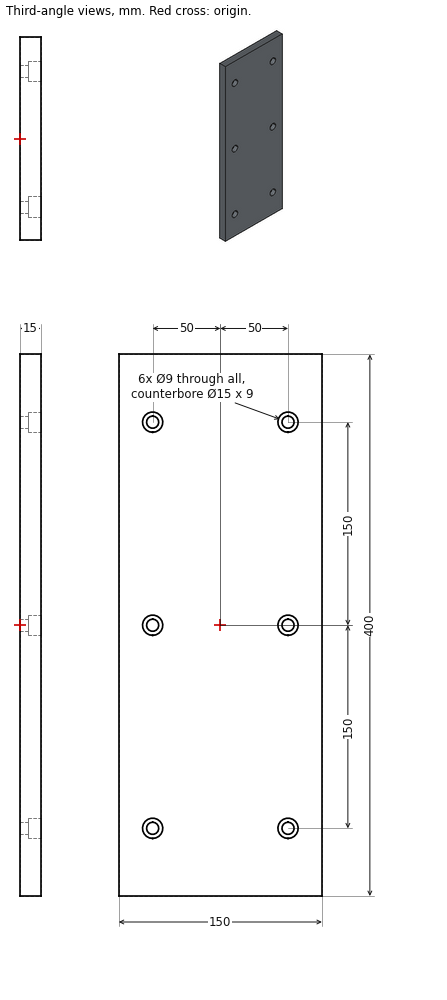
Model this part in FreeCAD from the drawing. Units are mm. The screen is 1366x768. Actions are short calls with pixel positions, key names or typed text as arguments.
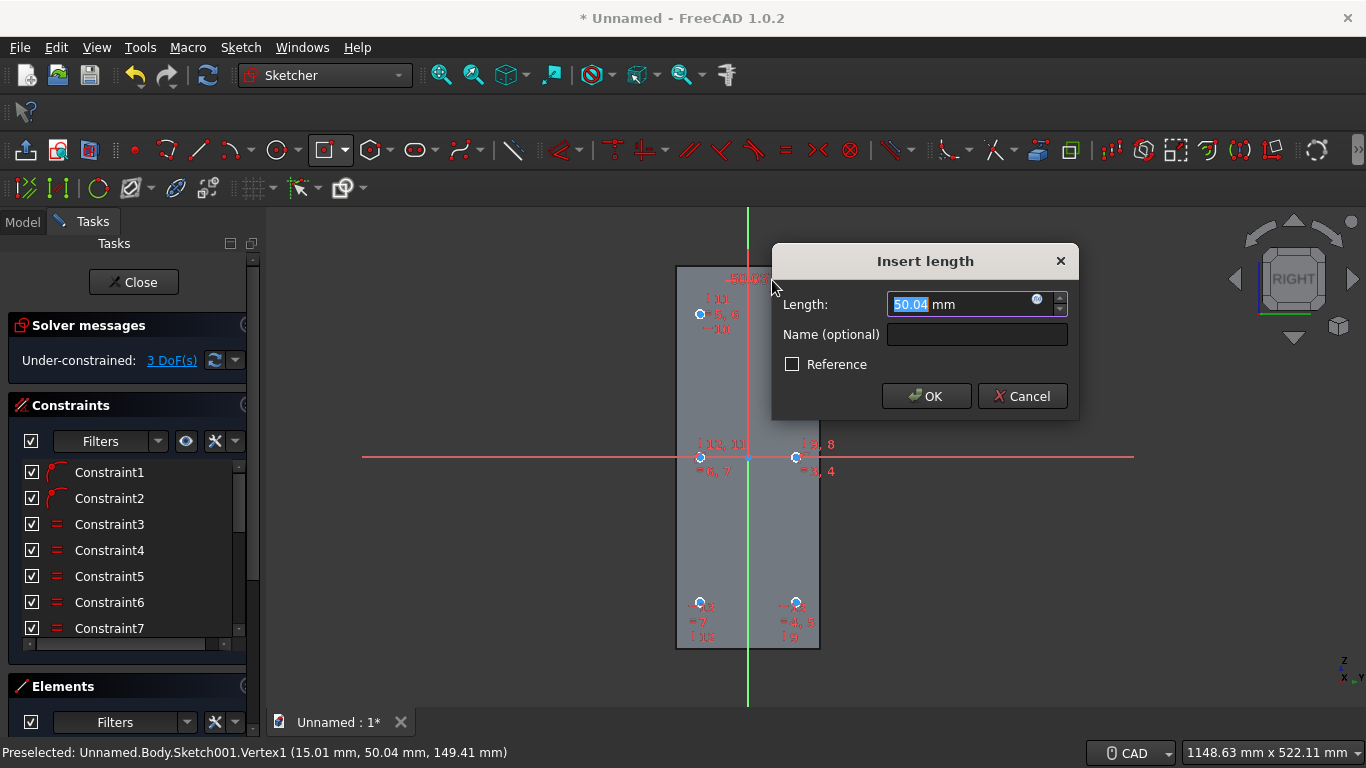
text(50)
key(Return)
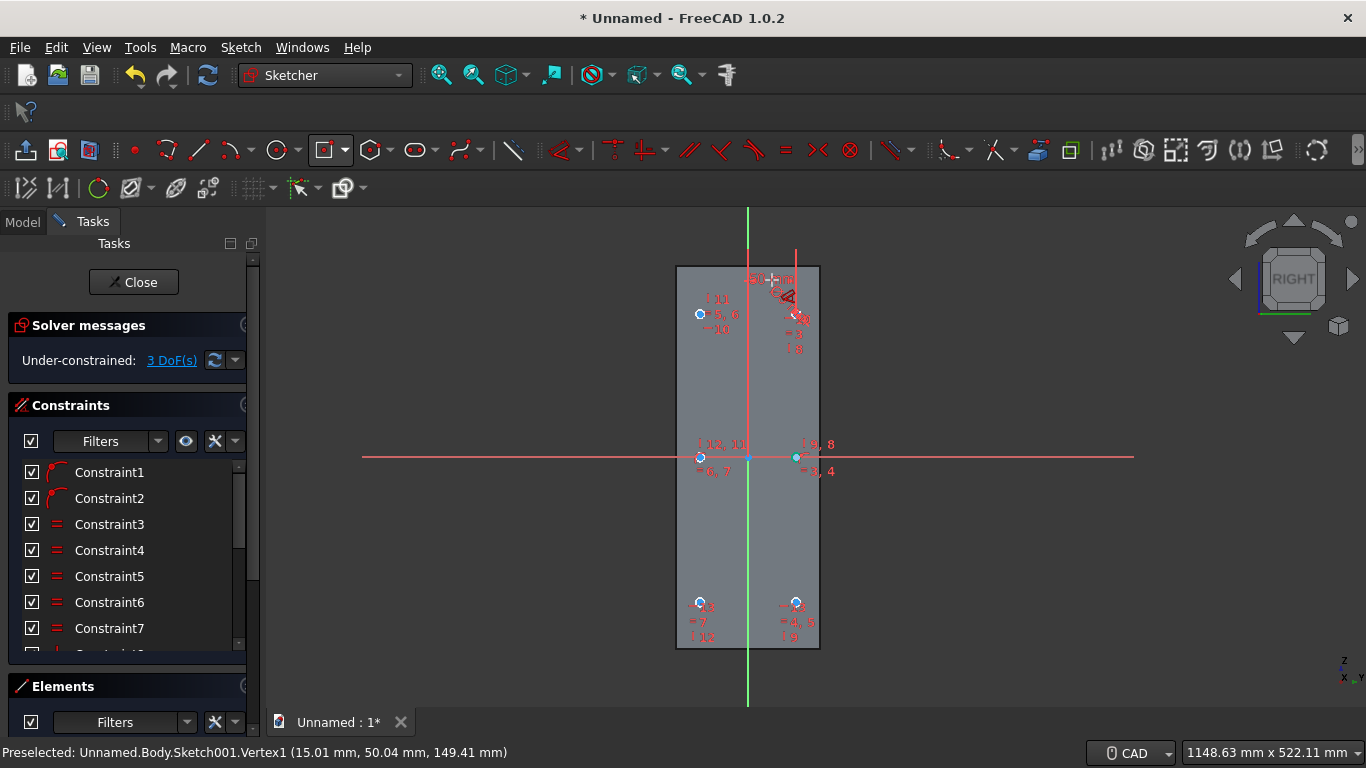
click(700, 314)
click(724, 491)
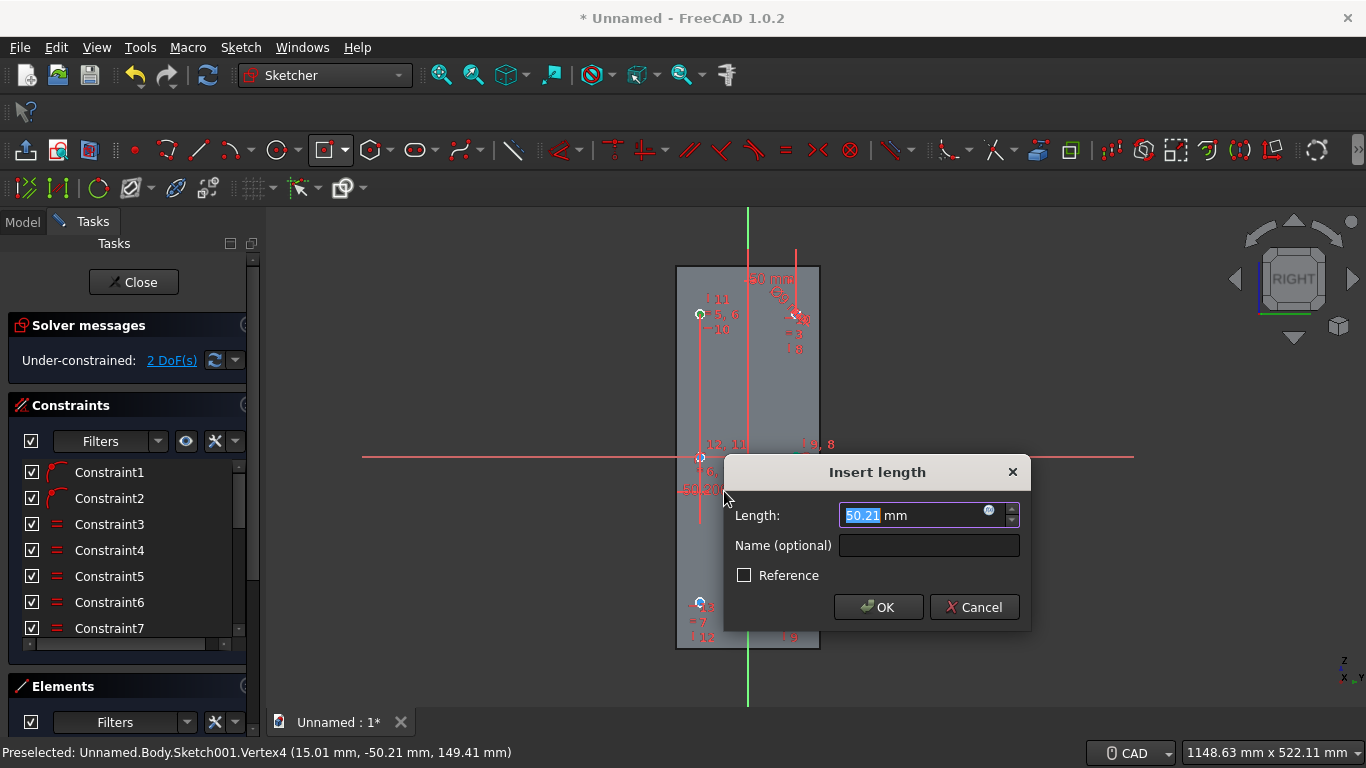
text(50)
key(Return)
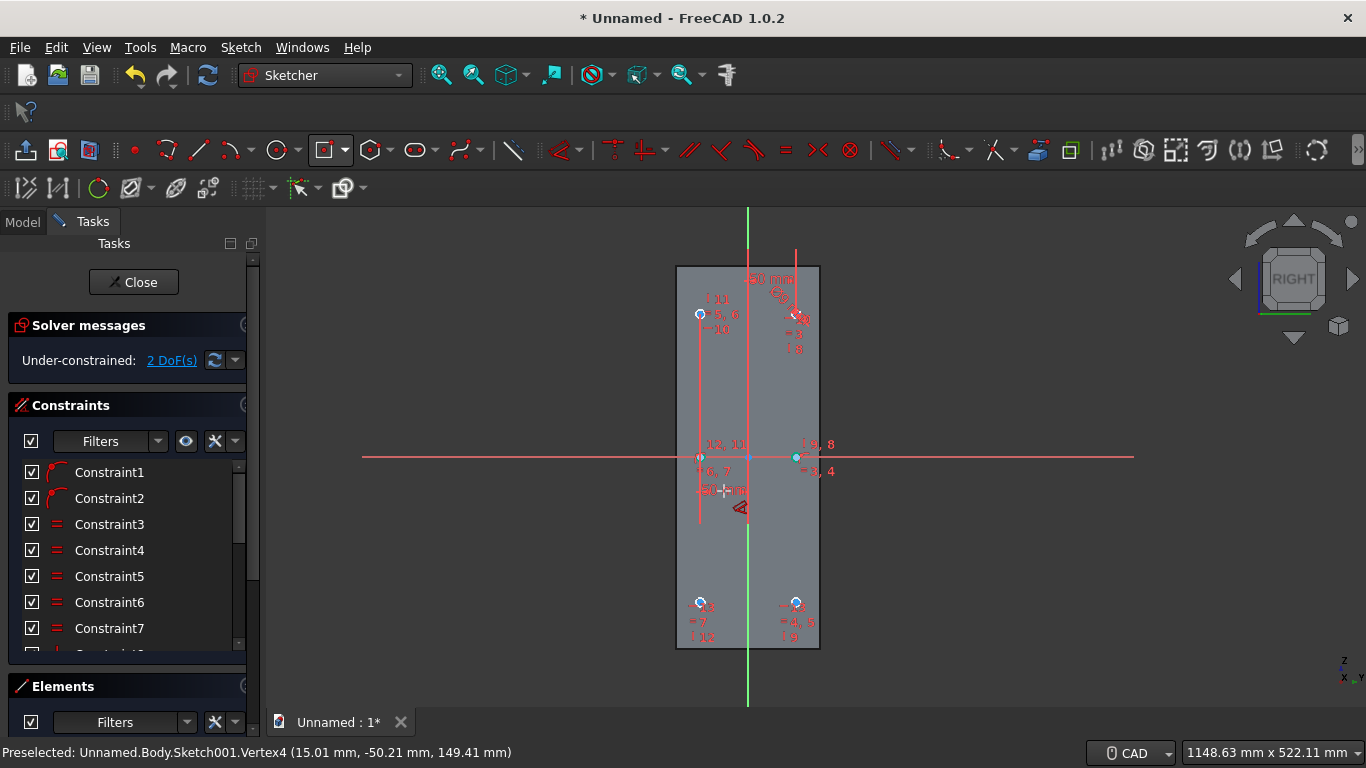
click(796, 314)
click(830, 386)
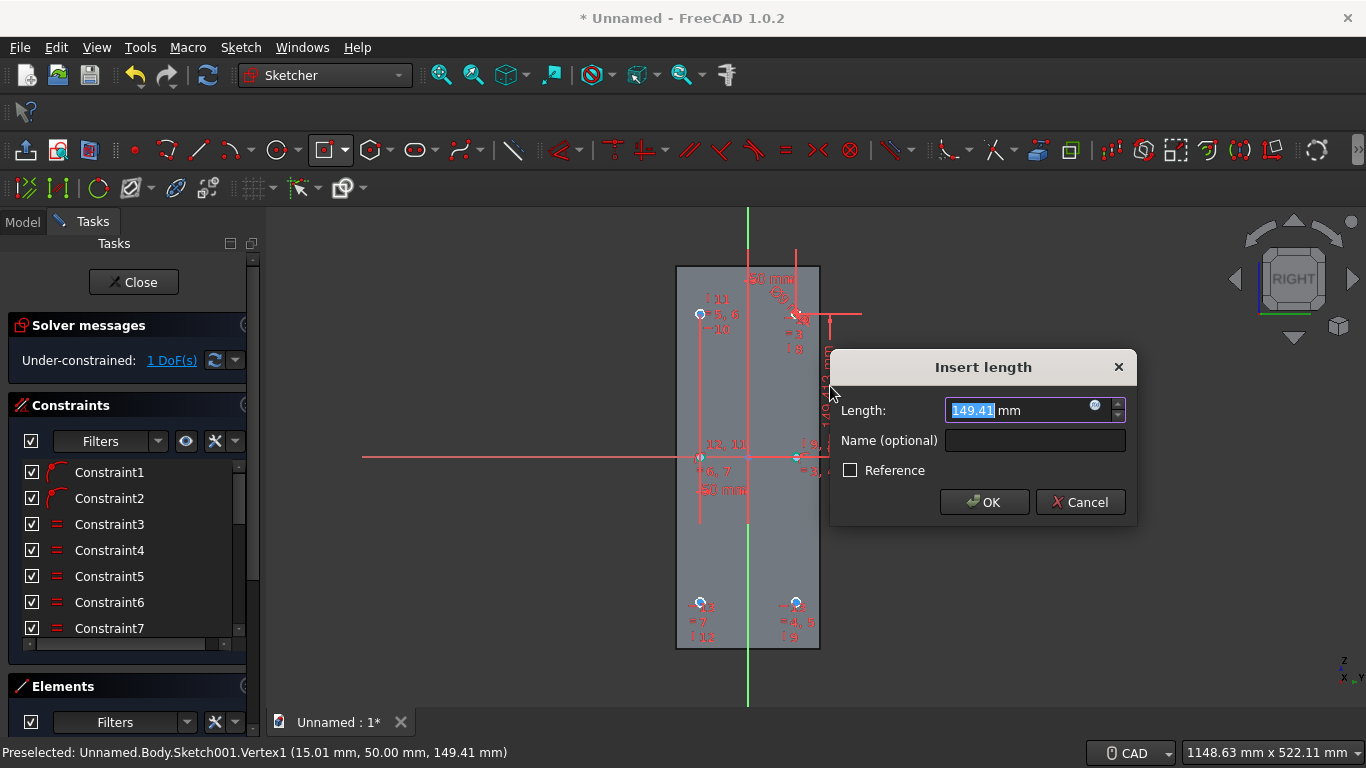
text(150)
key(Return)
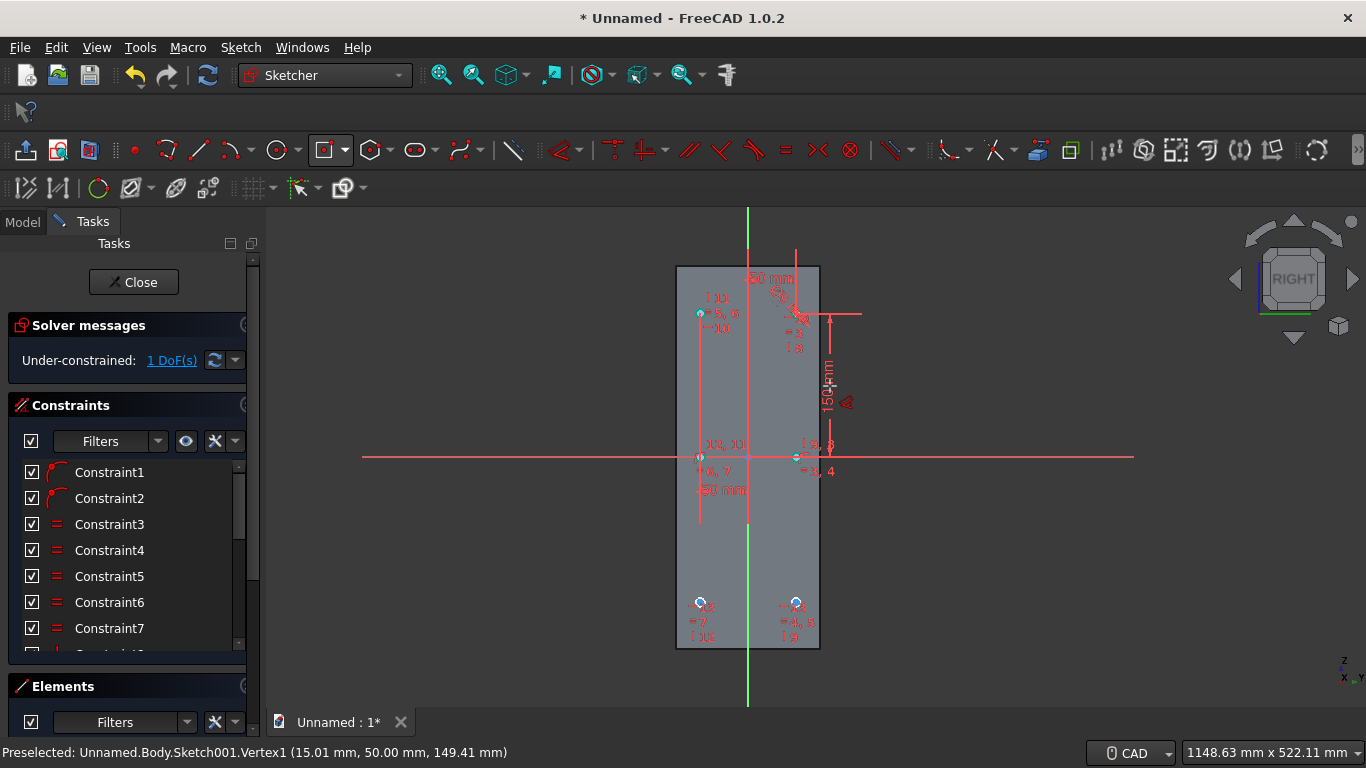
click(796, 602)
click(830, 530)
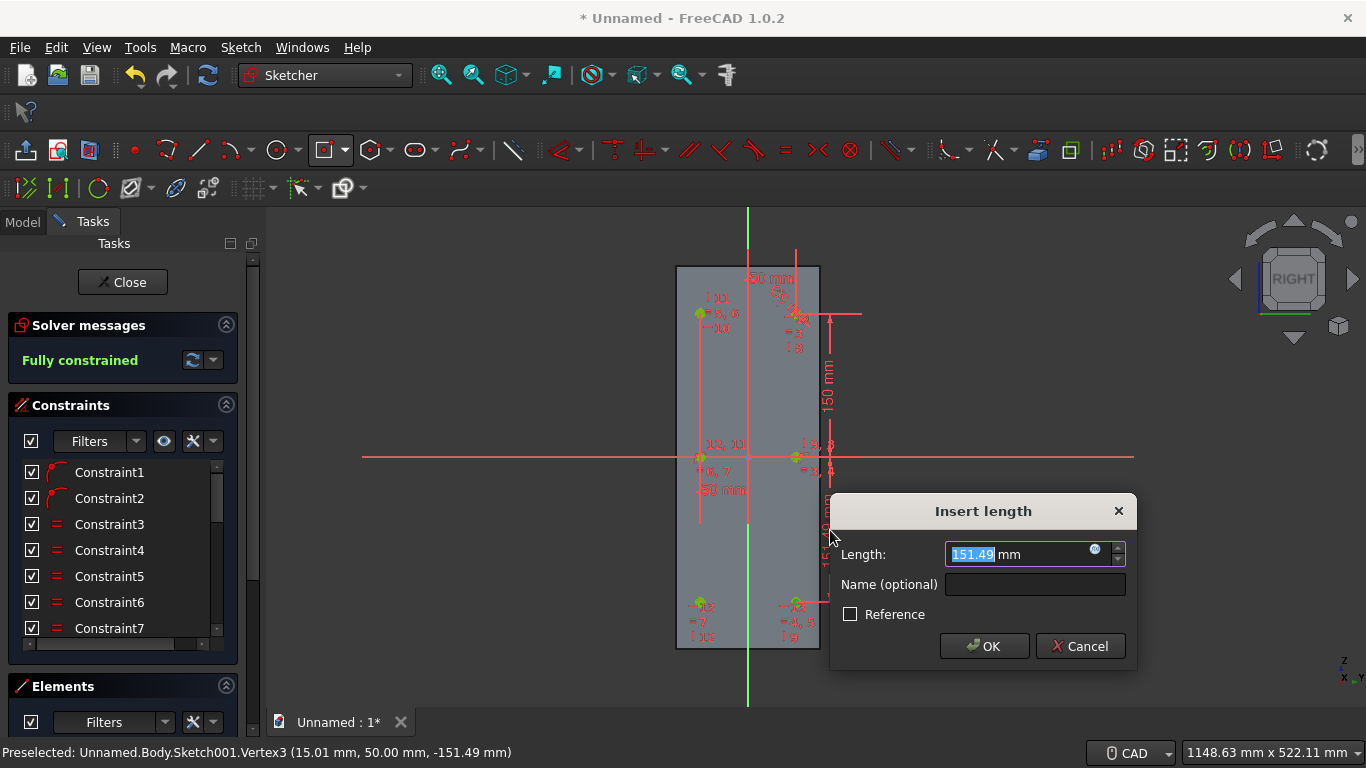
text(150)
key(Return)
key(Escape)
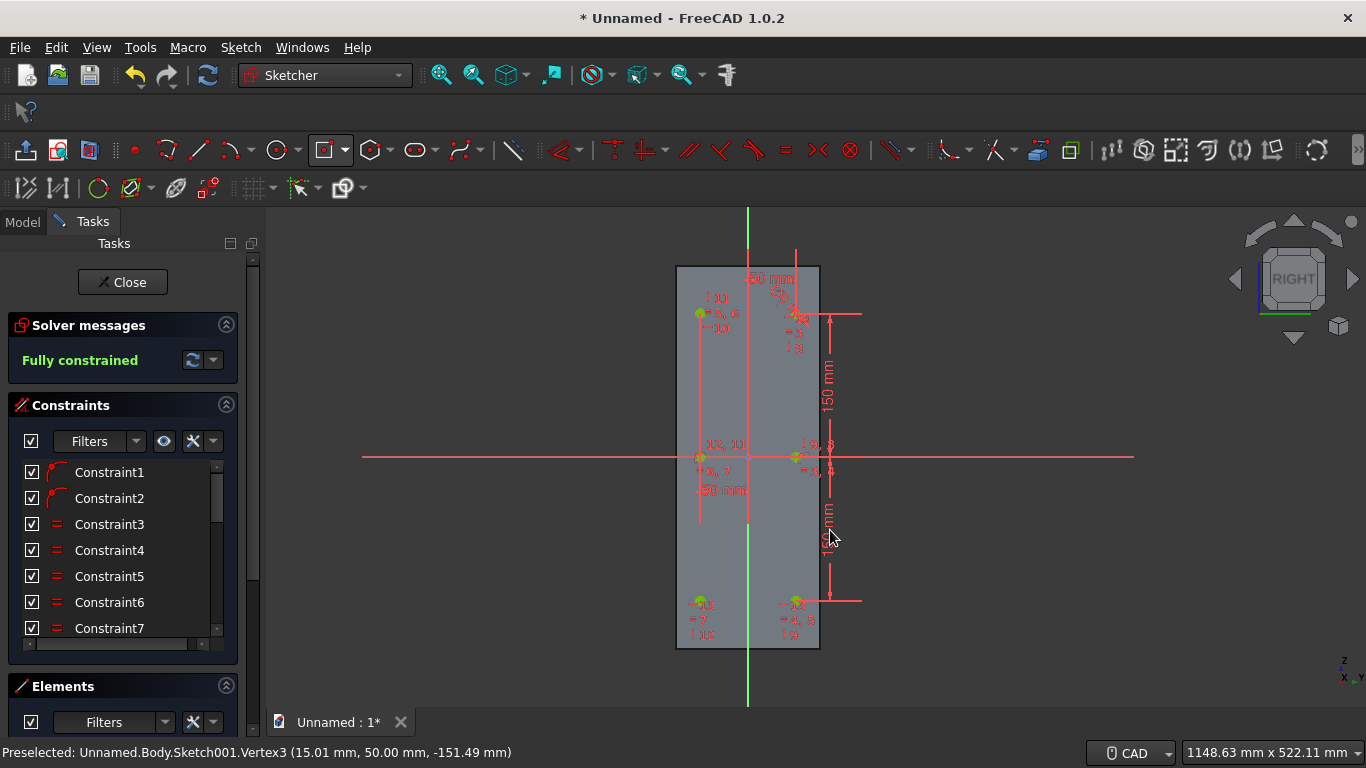
click(123, 282)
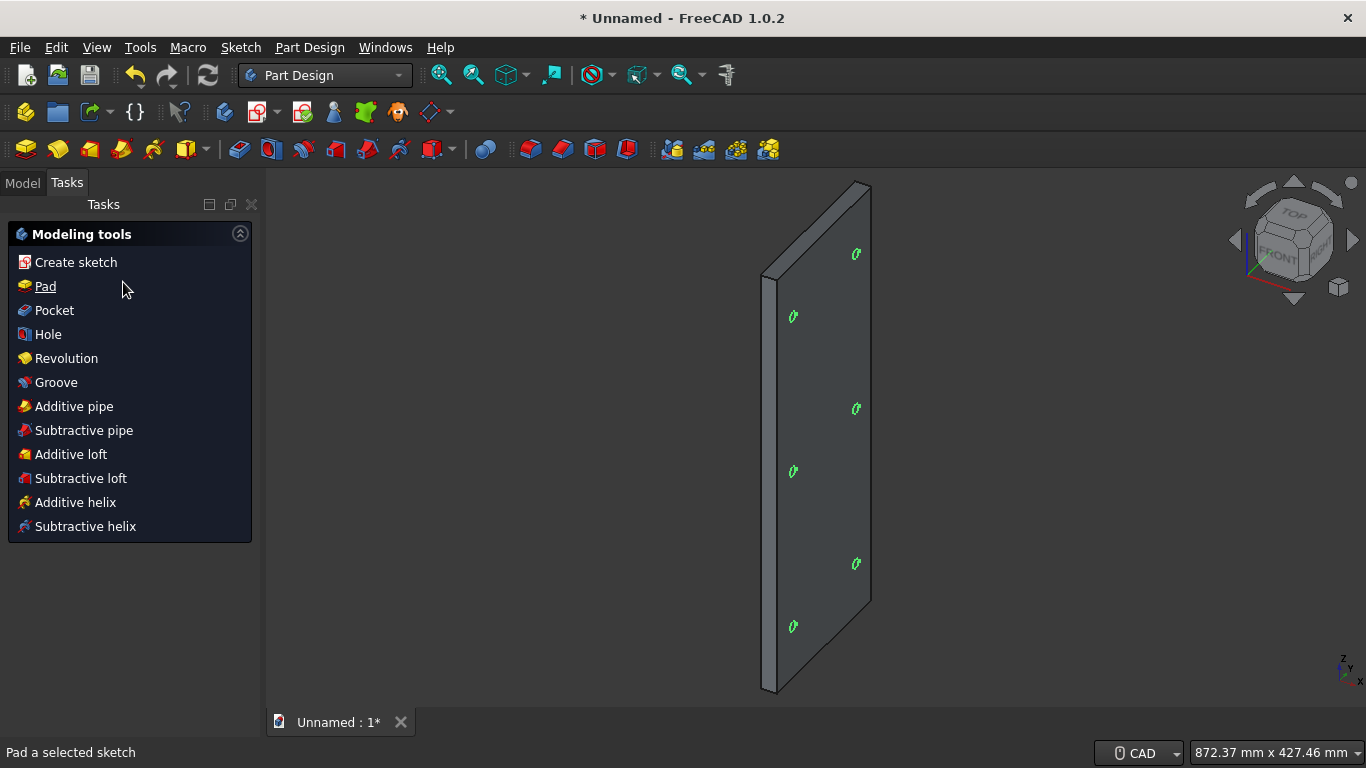
click(272, 150)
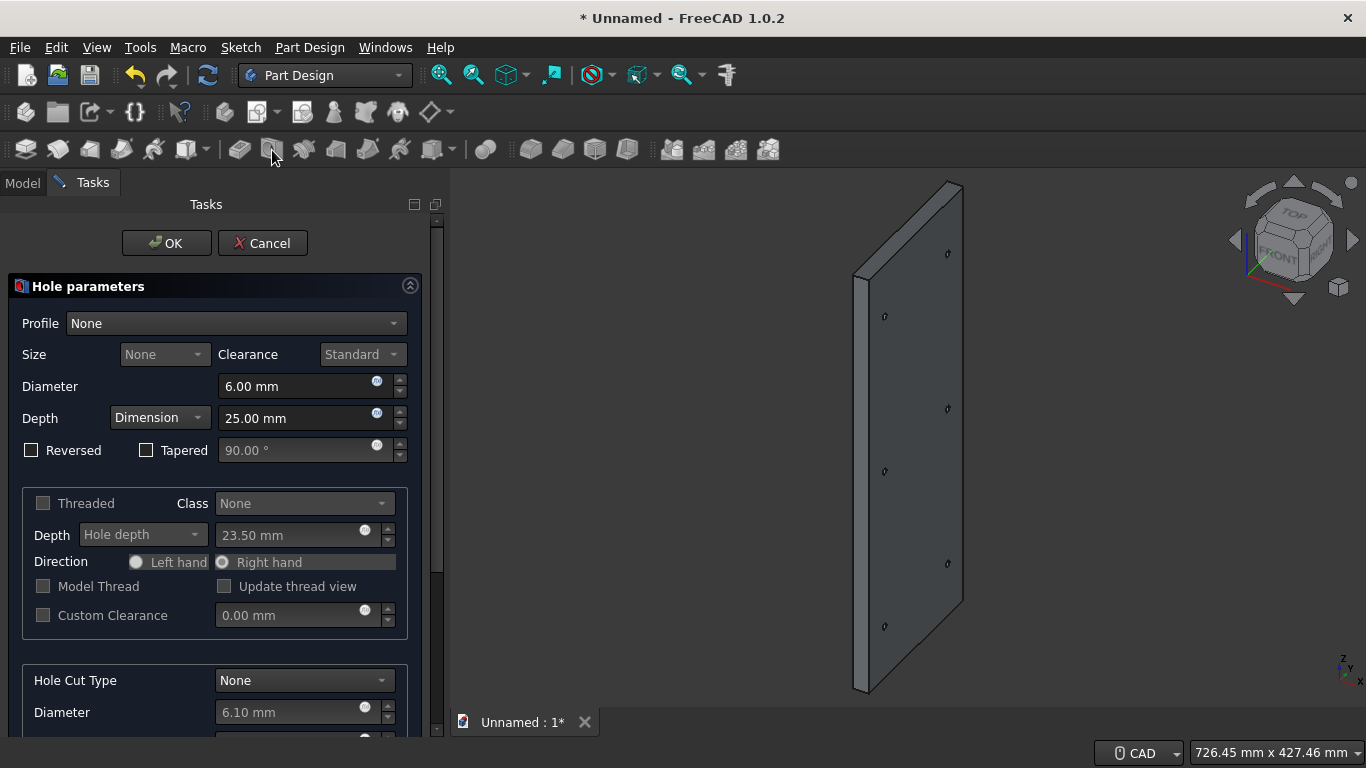
triple_click(305, 386)